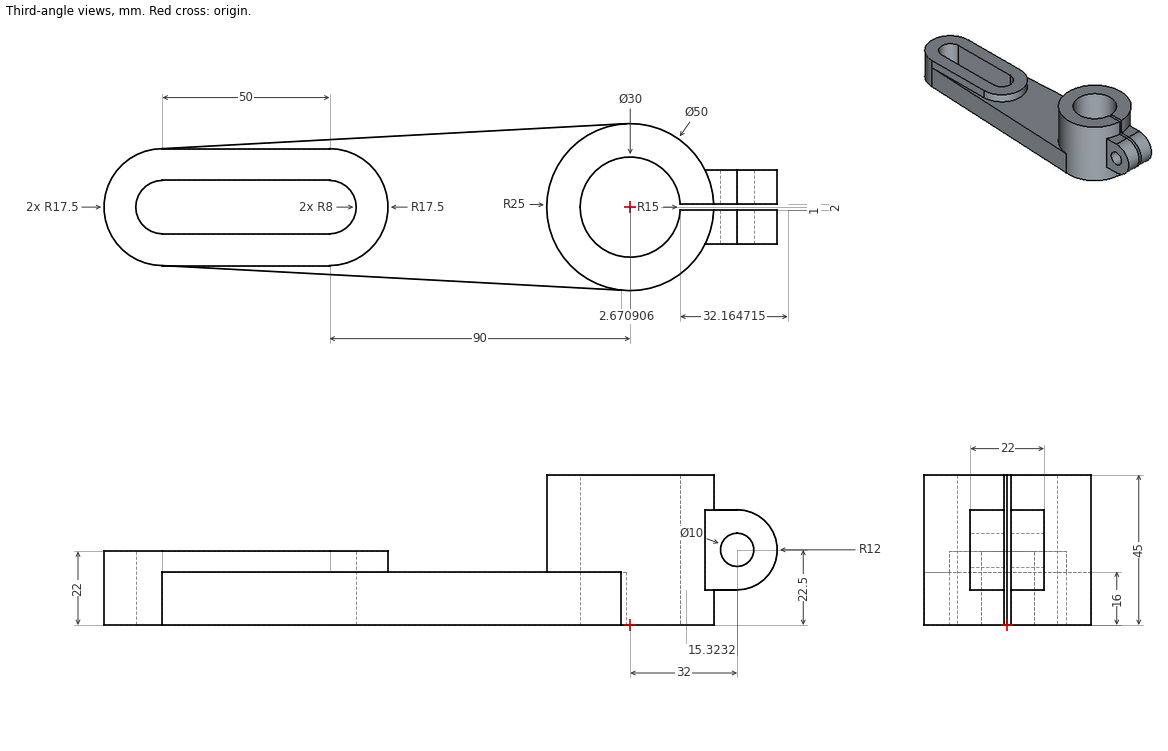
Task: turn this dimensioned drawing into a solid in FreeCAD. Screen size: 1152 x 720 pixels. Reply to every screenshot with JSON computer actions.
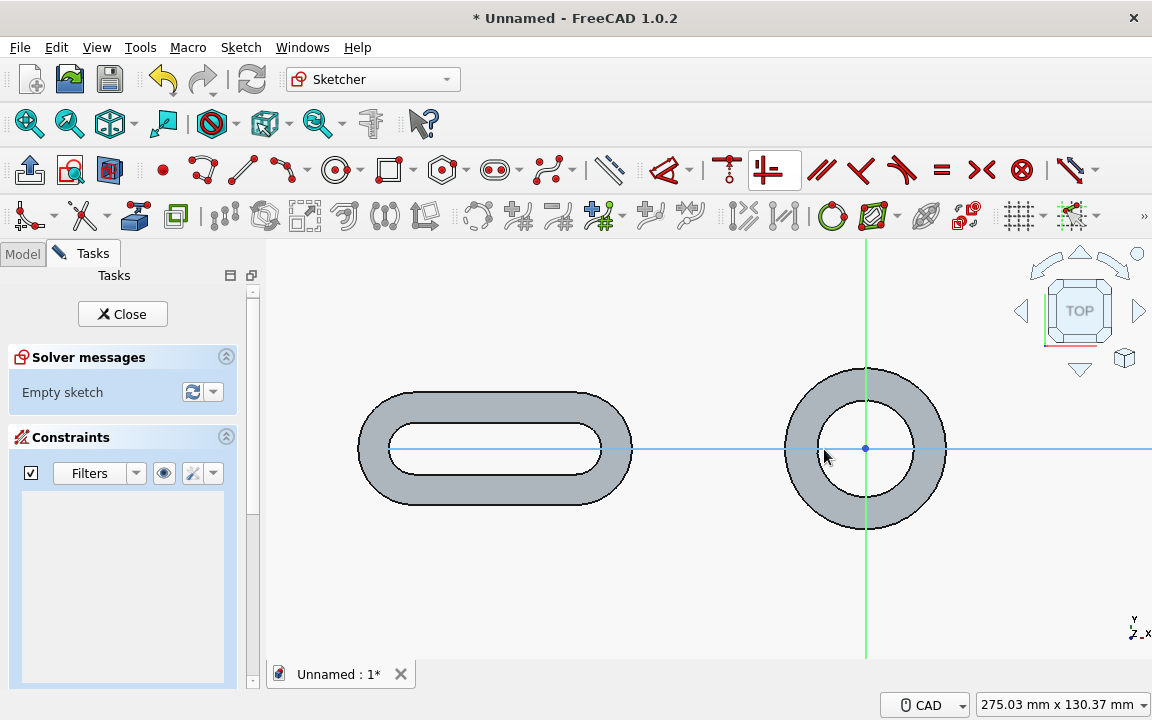
{"action": "left_click", "coordinate": [204, 170]}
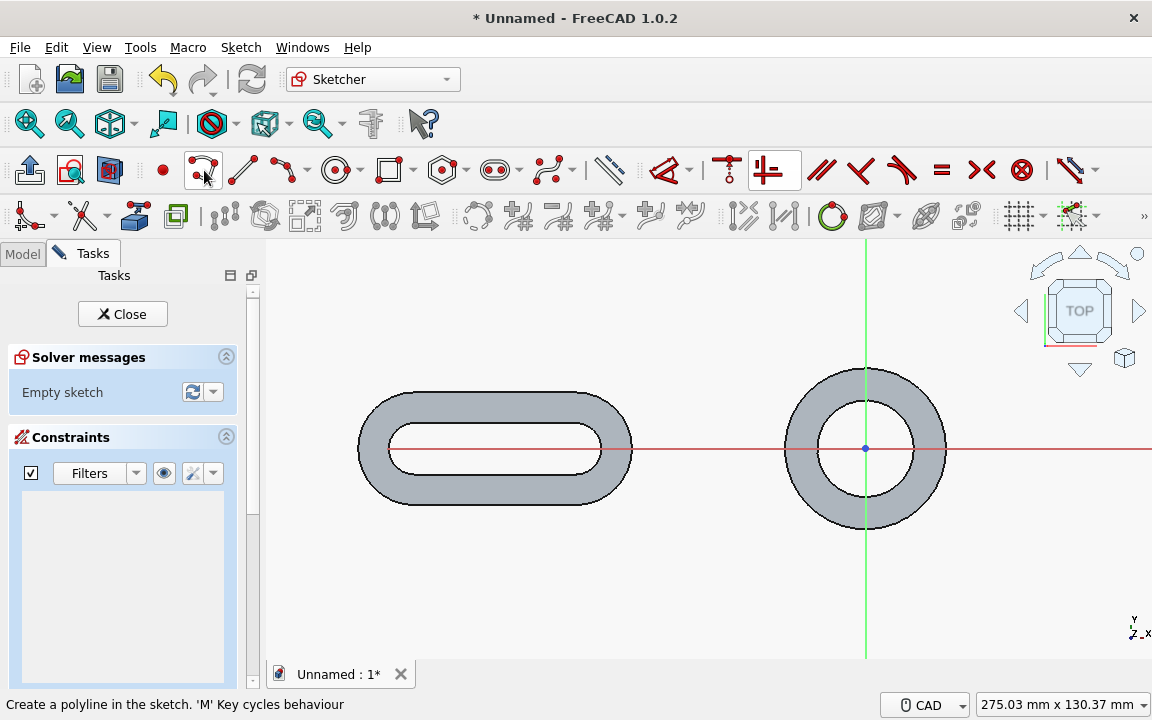
{"action": "scroll", "coordinate": [861, 368], "scroll_direction": "up", "scroll_amount": 7}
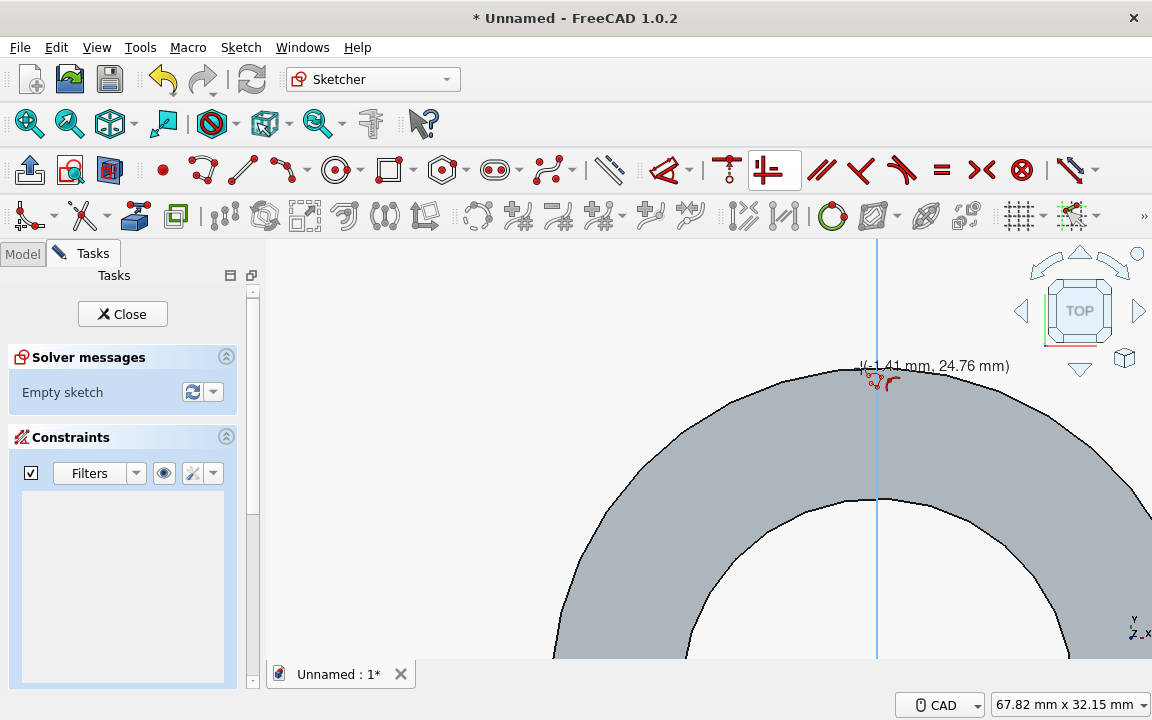
{"action": "left_click", "coordinate": [860, 368]}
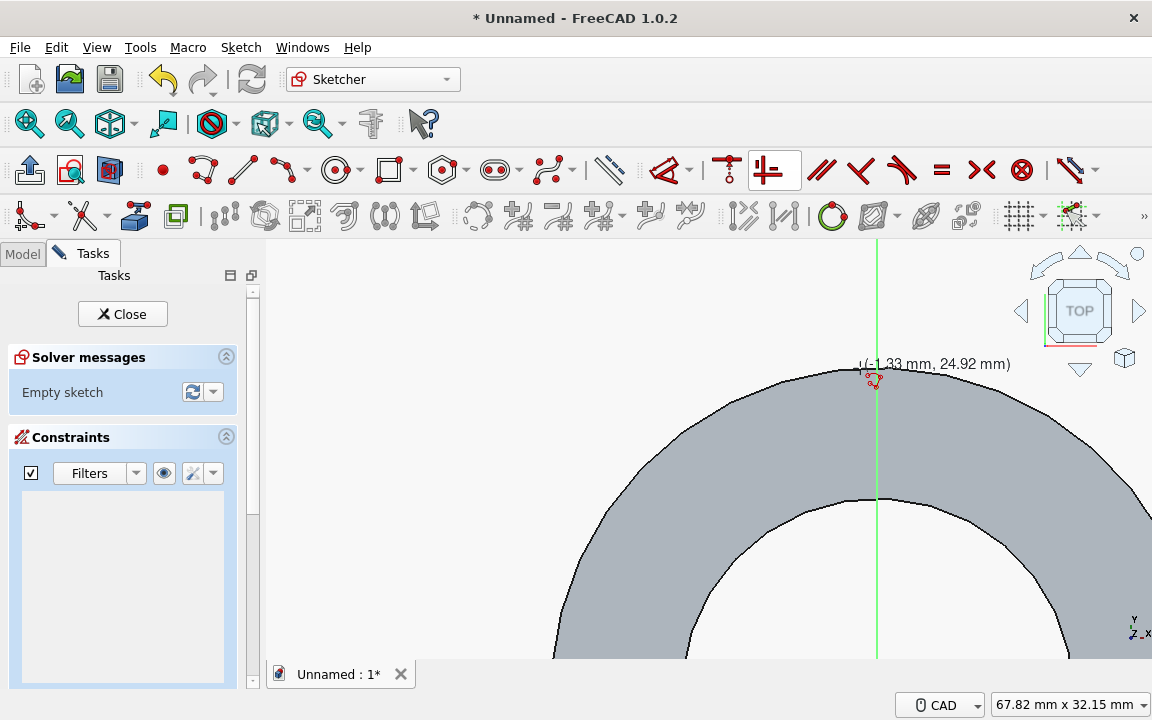
{"action": "scroll", "coordinate": [862, 369], "scroll_direction": "down", "scroll_amount": 7}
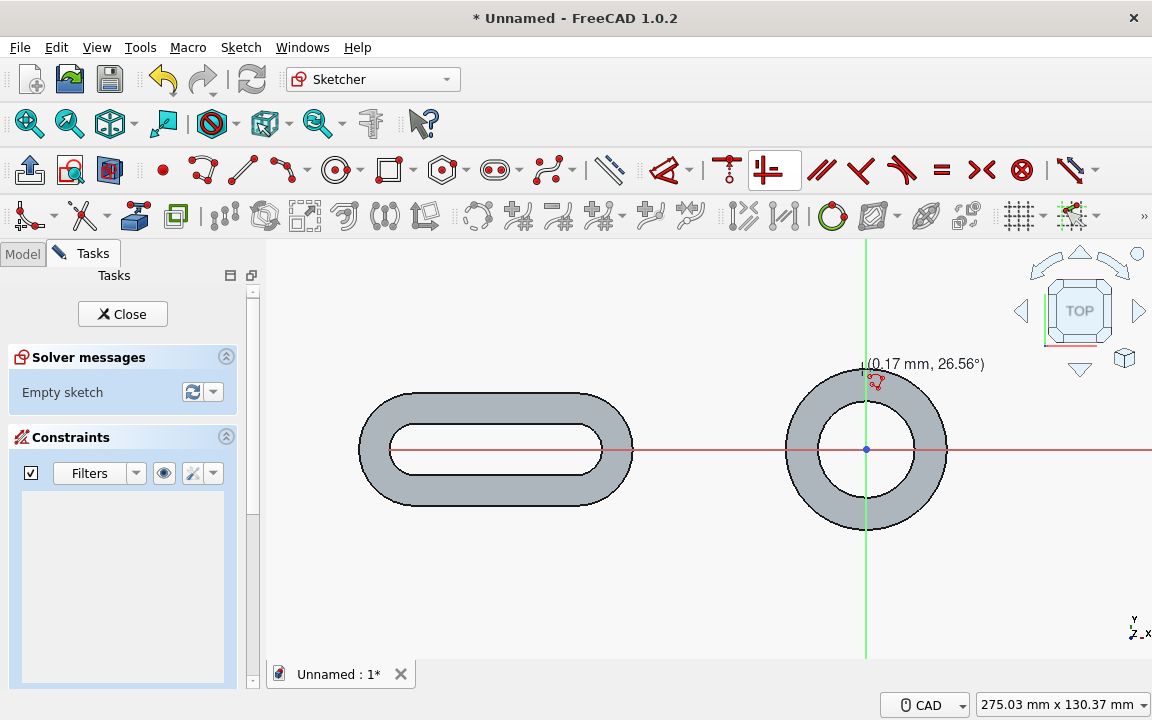
{"action": "left_click", "coordinate": [415, 393]}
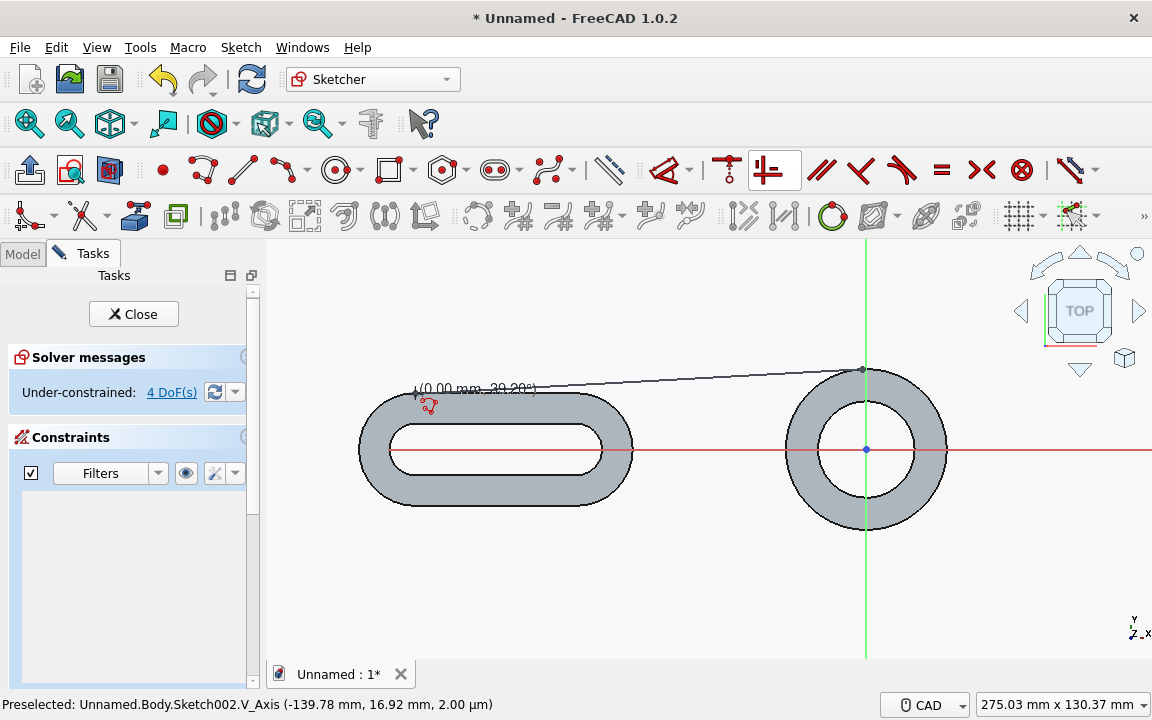
{"action": "scroll", "coordinate": [576, 393], "scroll_direction": "up", "scroll_amount": 4}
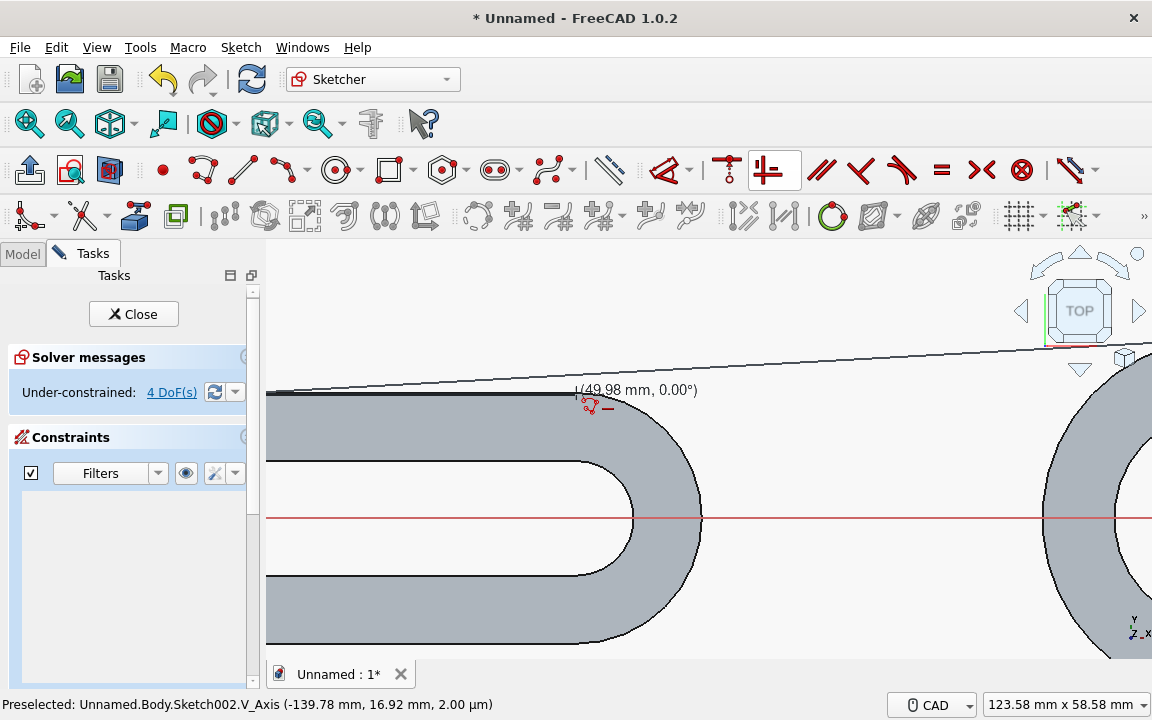
{"action": "left_click", "coordinate": [576, 393]}
{"action": "right_click", "coordinate": [576, 393]}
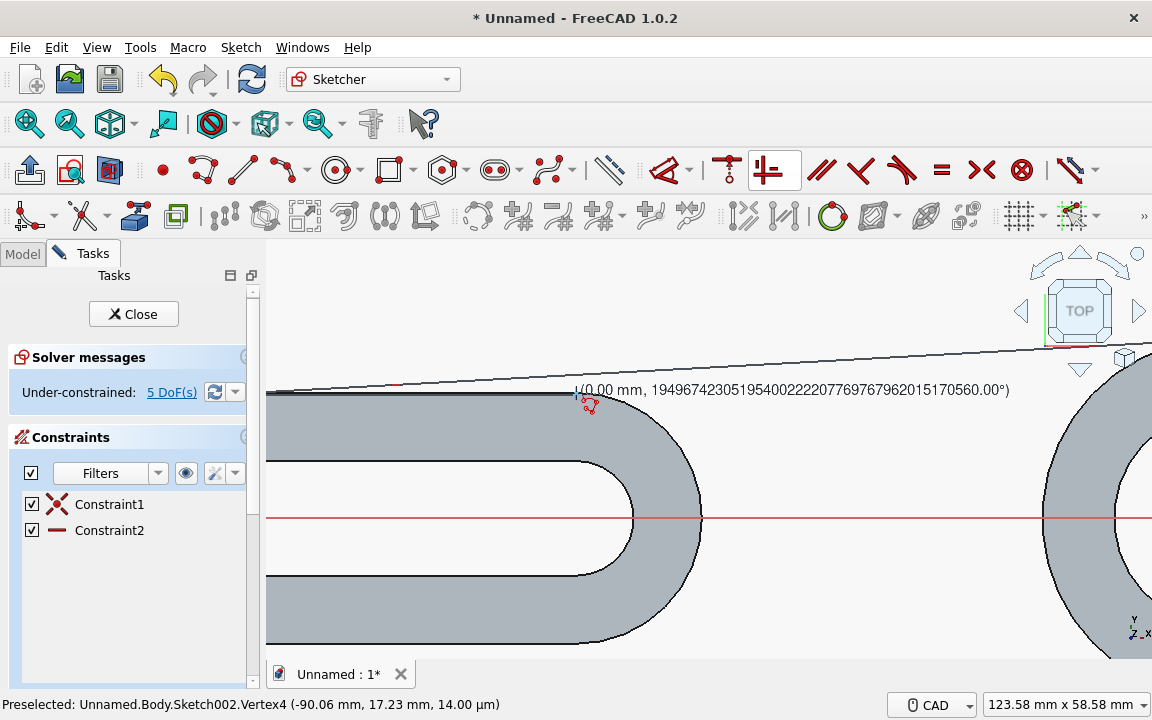
{"action": "scroll", "coordinate": [576, 393], "scroll_direction": "down", "scroll_amount": 4}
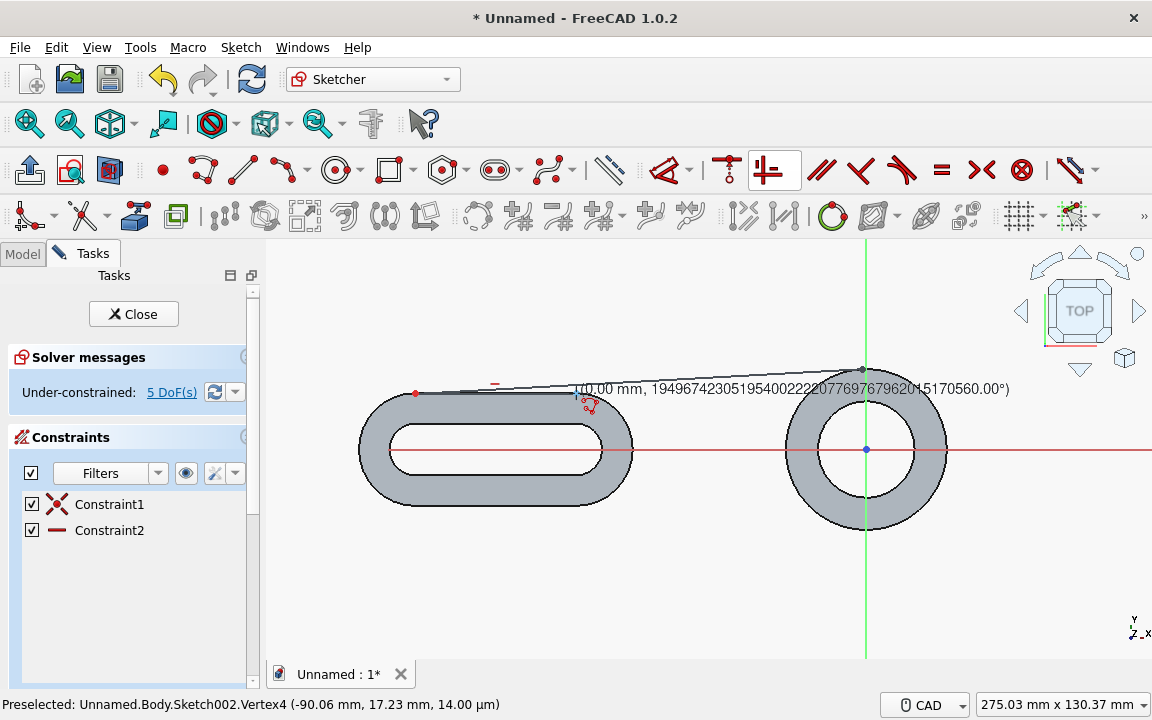
{"action": "left_click", "coordinate": [576, 506]}
{"action": "left_click", "coordinate": [415, 506]}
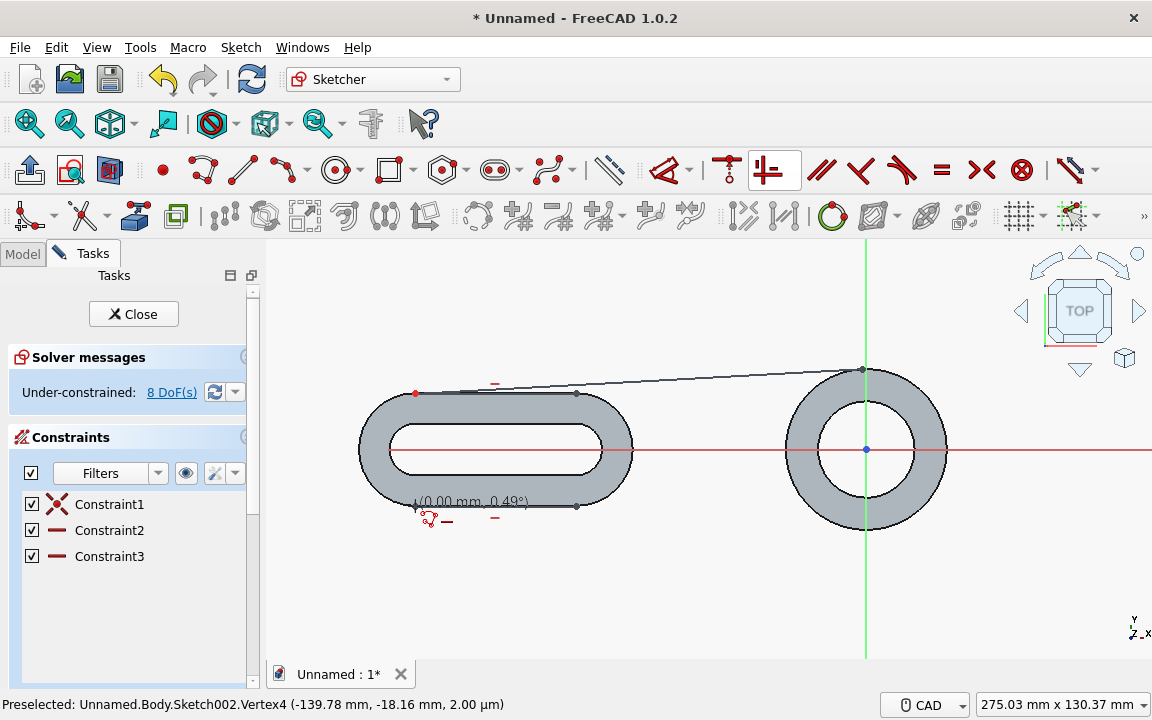
{"action": "scroll", "coordinate": [858, 530], "scroll_direction": "up", "scroll_amount": 4}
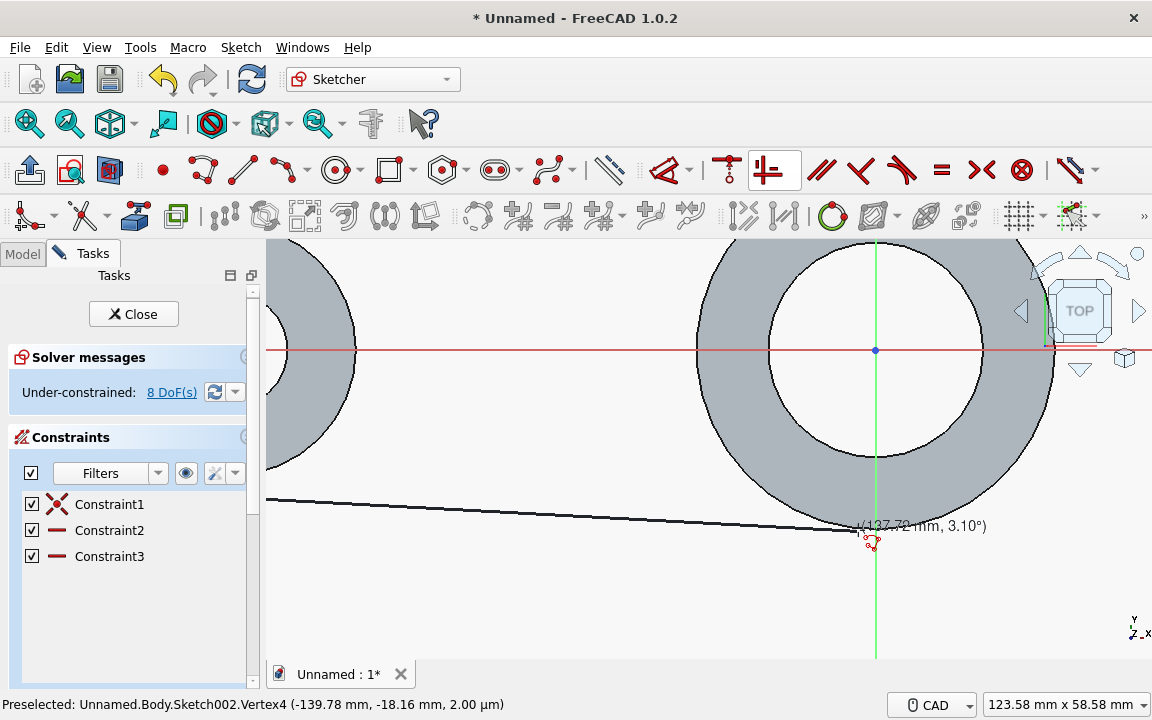
{"action": "left_click", "coordinate": [857, 528]}
{"action": "right_click", "coordinate": [857, 528]}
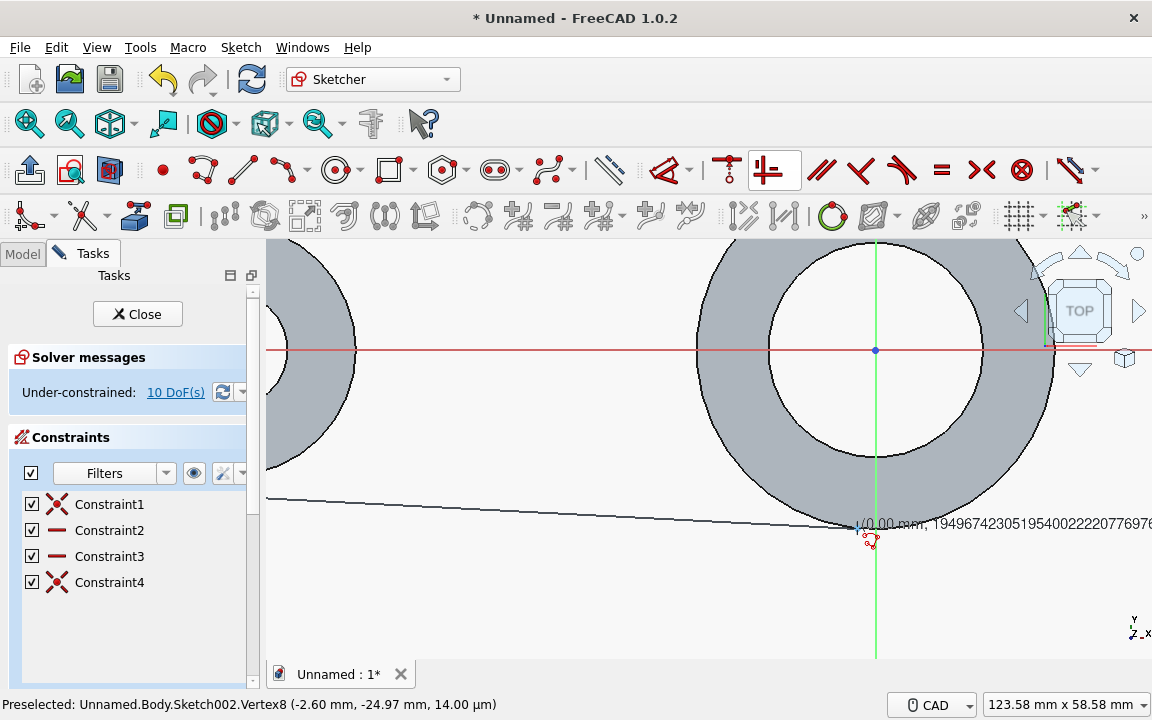
{"action": "key", "text": "g 3 a"}